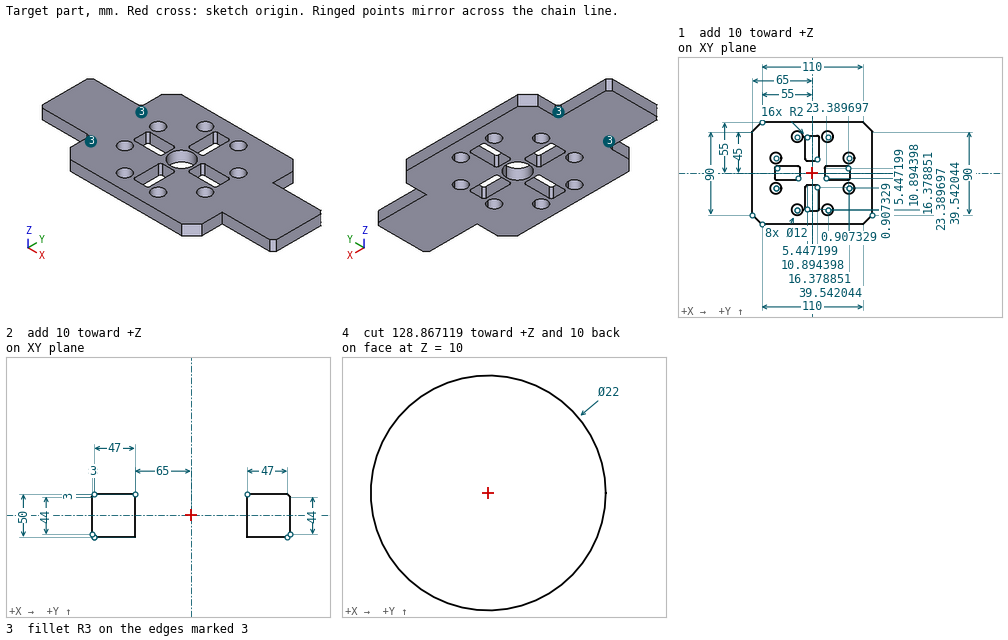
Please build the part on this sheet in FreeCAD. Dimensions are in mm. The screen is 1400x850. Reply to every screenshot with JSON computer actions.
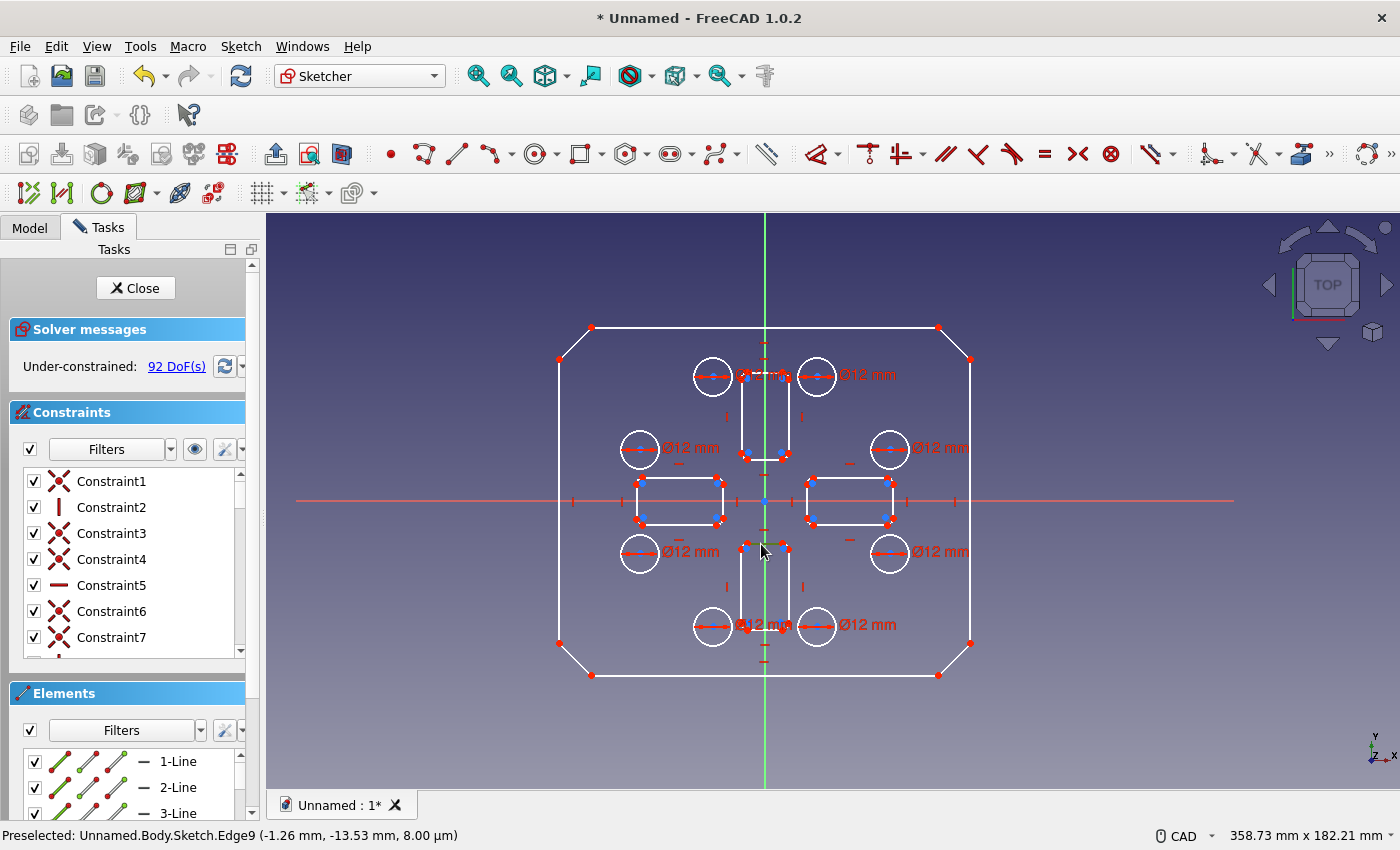
{"action": "scroll", "coordinate": [787, 545], "scroll_direction": "up", "scroll_amount": 6}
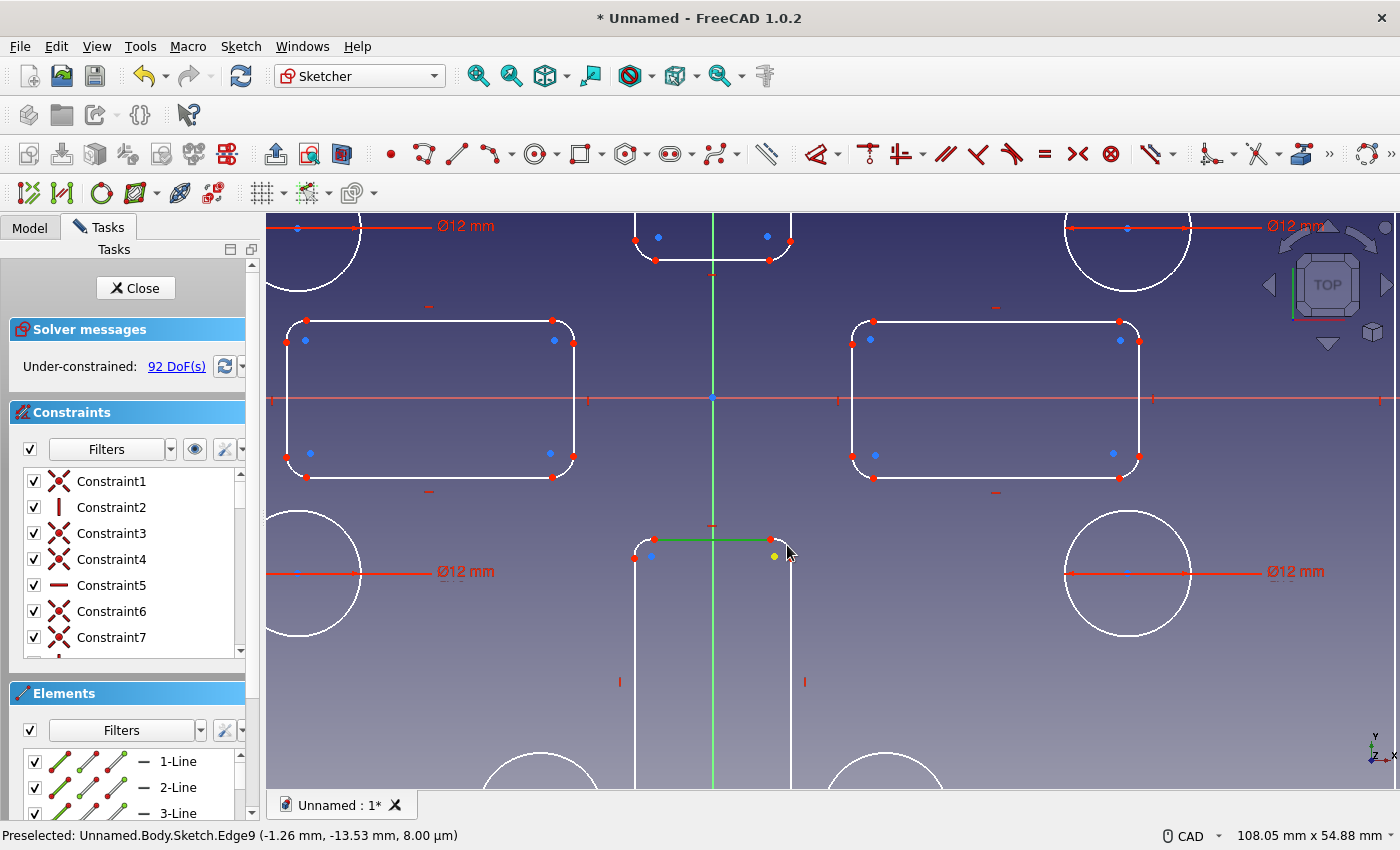
{"action": "left_click", "coordinate": [786, 544]}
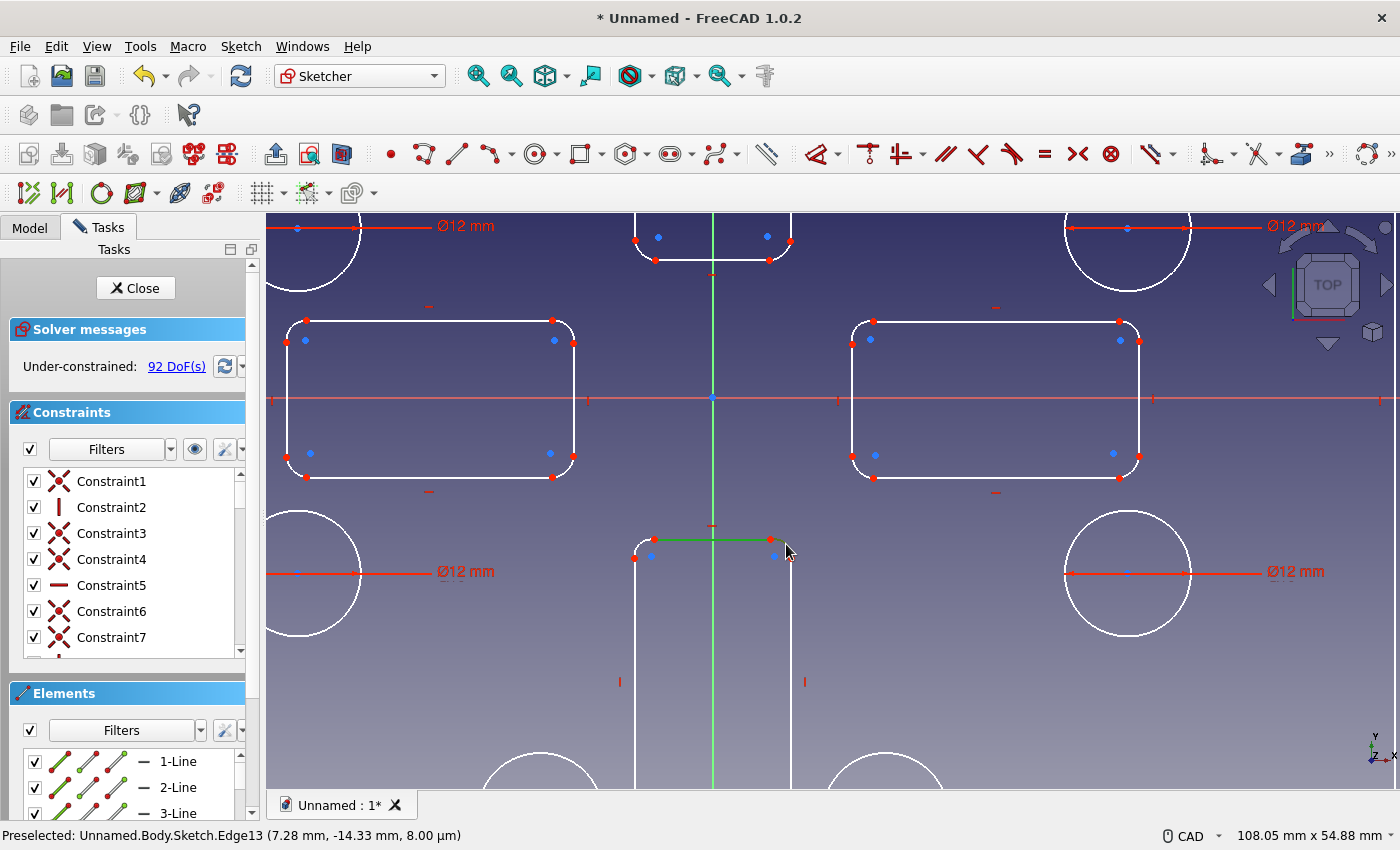
{"action": "left_click", "coordinate": [1012, 154]}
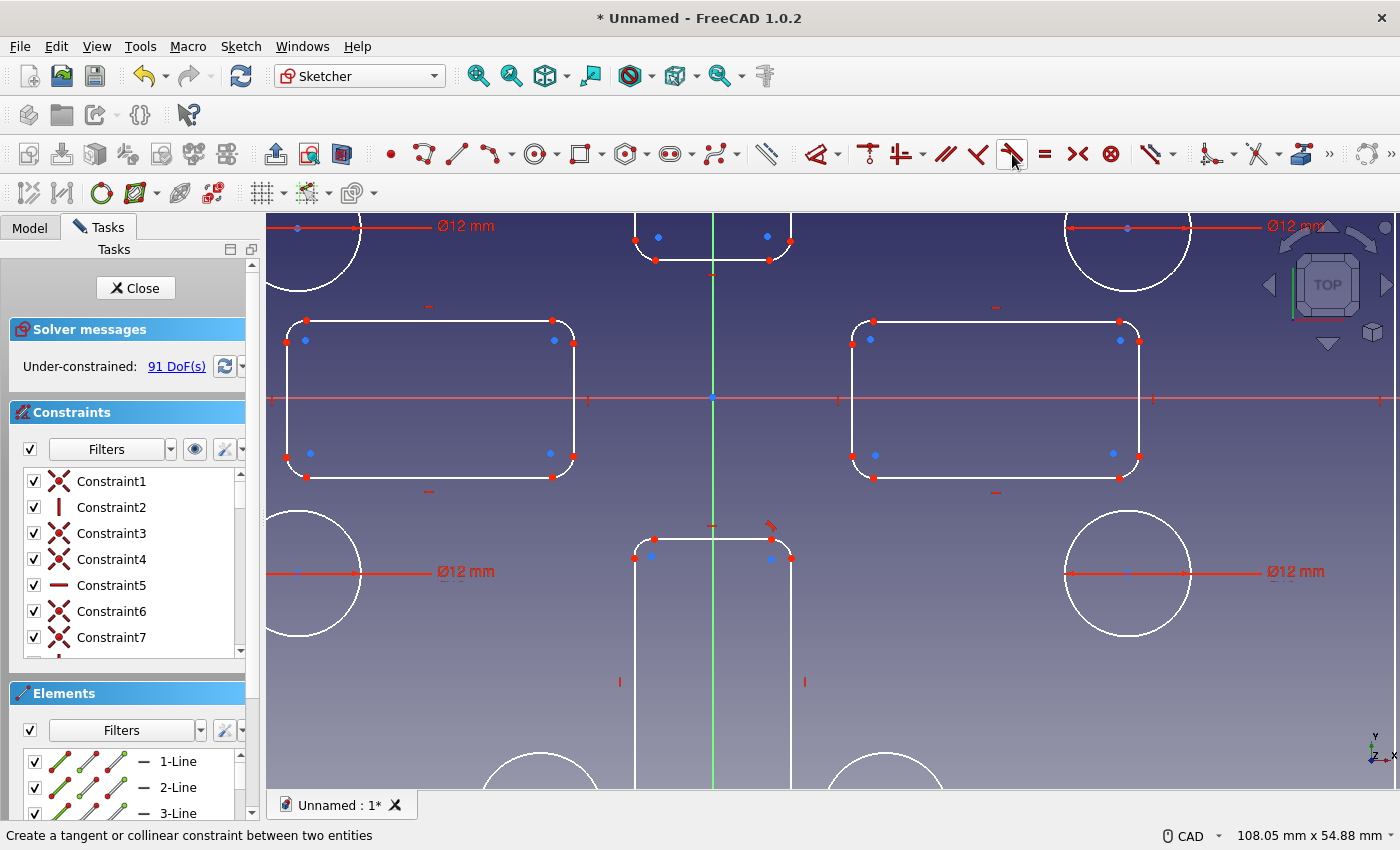
{"action": "left_click", "coordinate": [689, 539]}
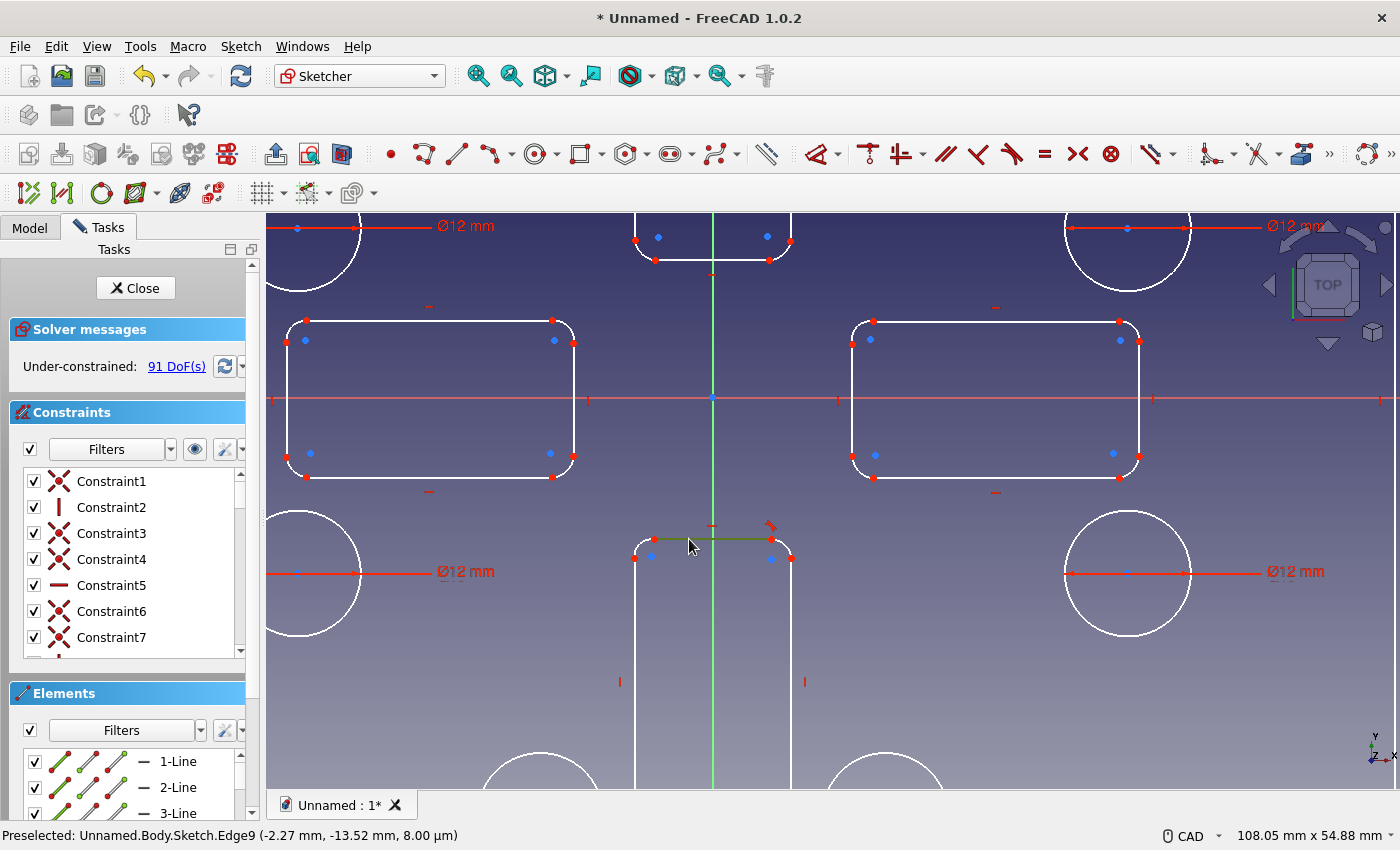
{"action": "scroll", "coordinate": [645, 541], "scroll_direction": "up", "scroll_amount": 2}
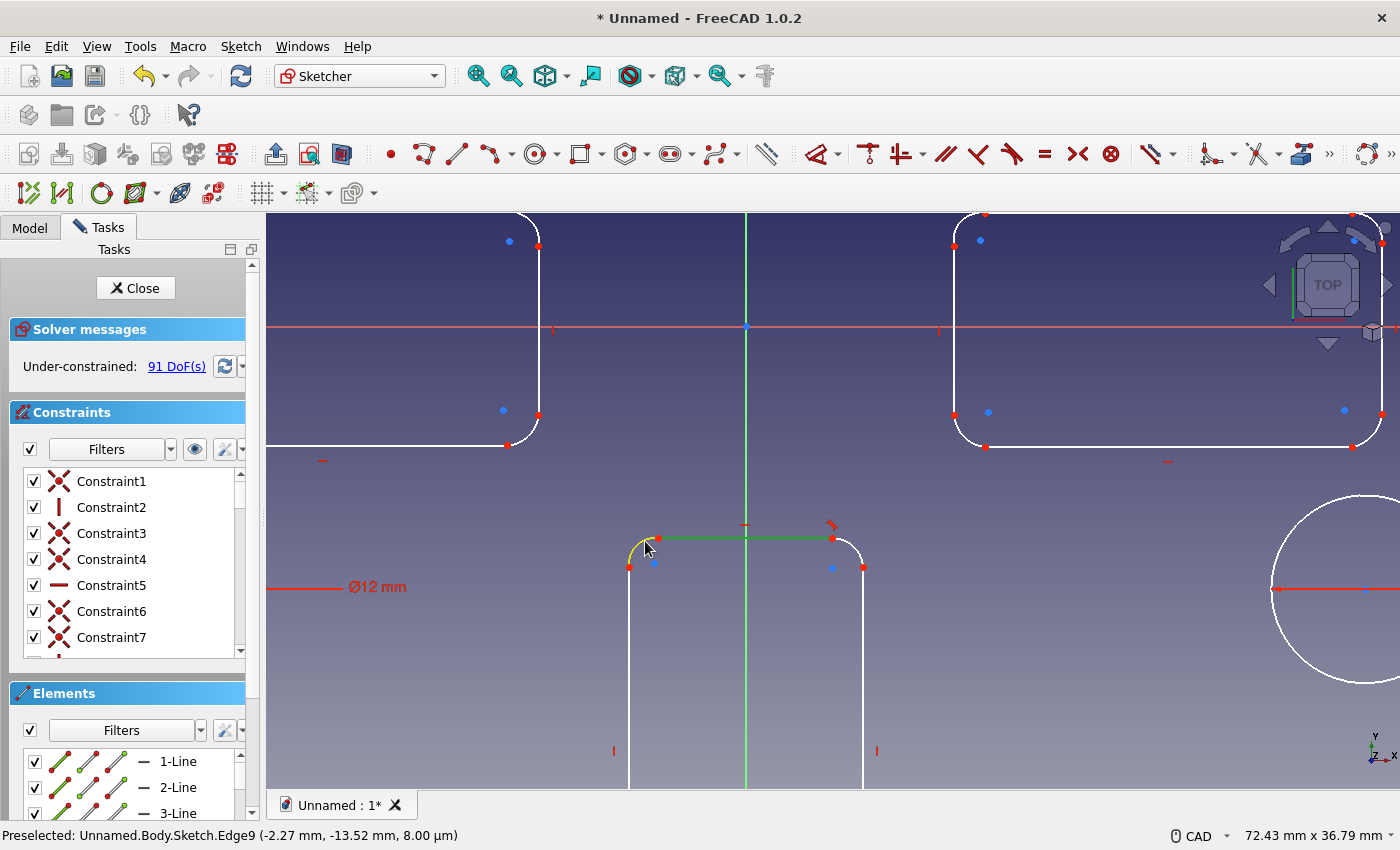
{"action": "left_click", "coordinate": [645, 540]}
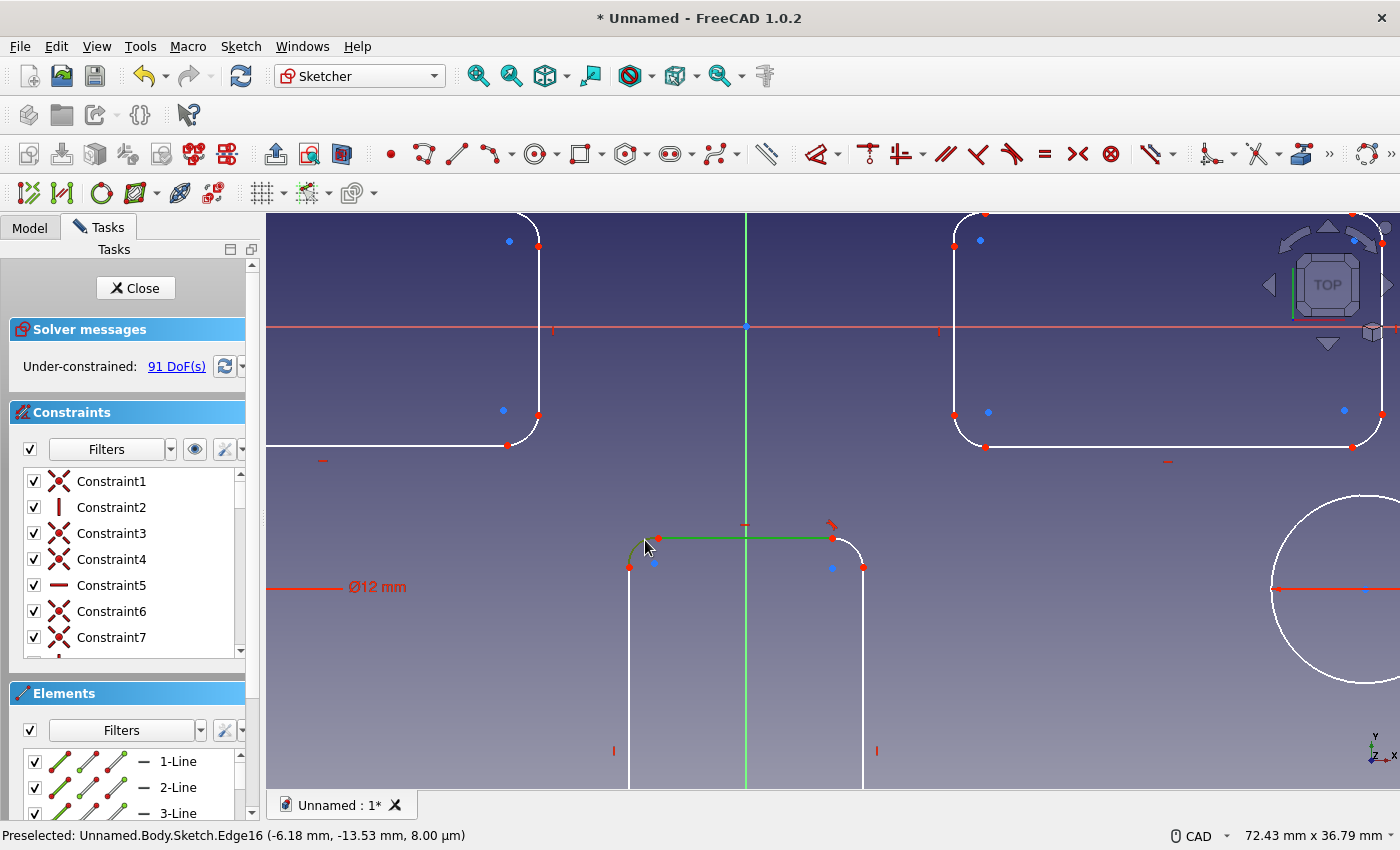
{"action": "left_click", "coordinate": [1012, 154]}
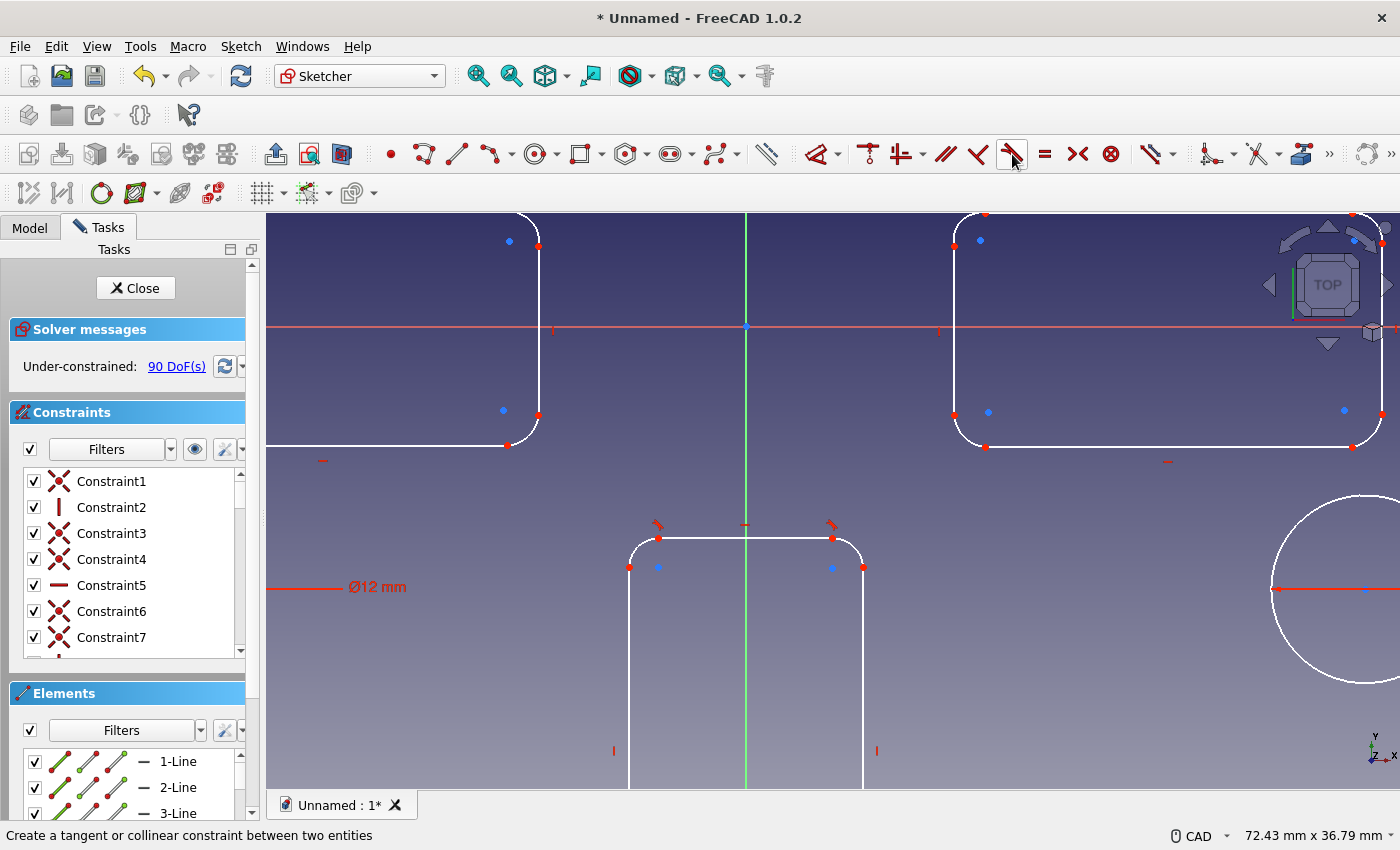
{"action": "scroll", "coordinate": [769, 545], "scroll_direction": "down", "scroll_amount": 8}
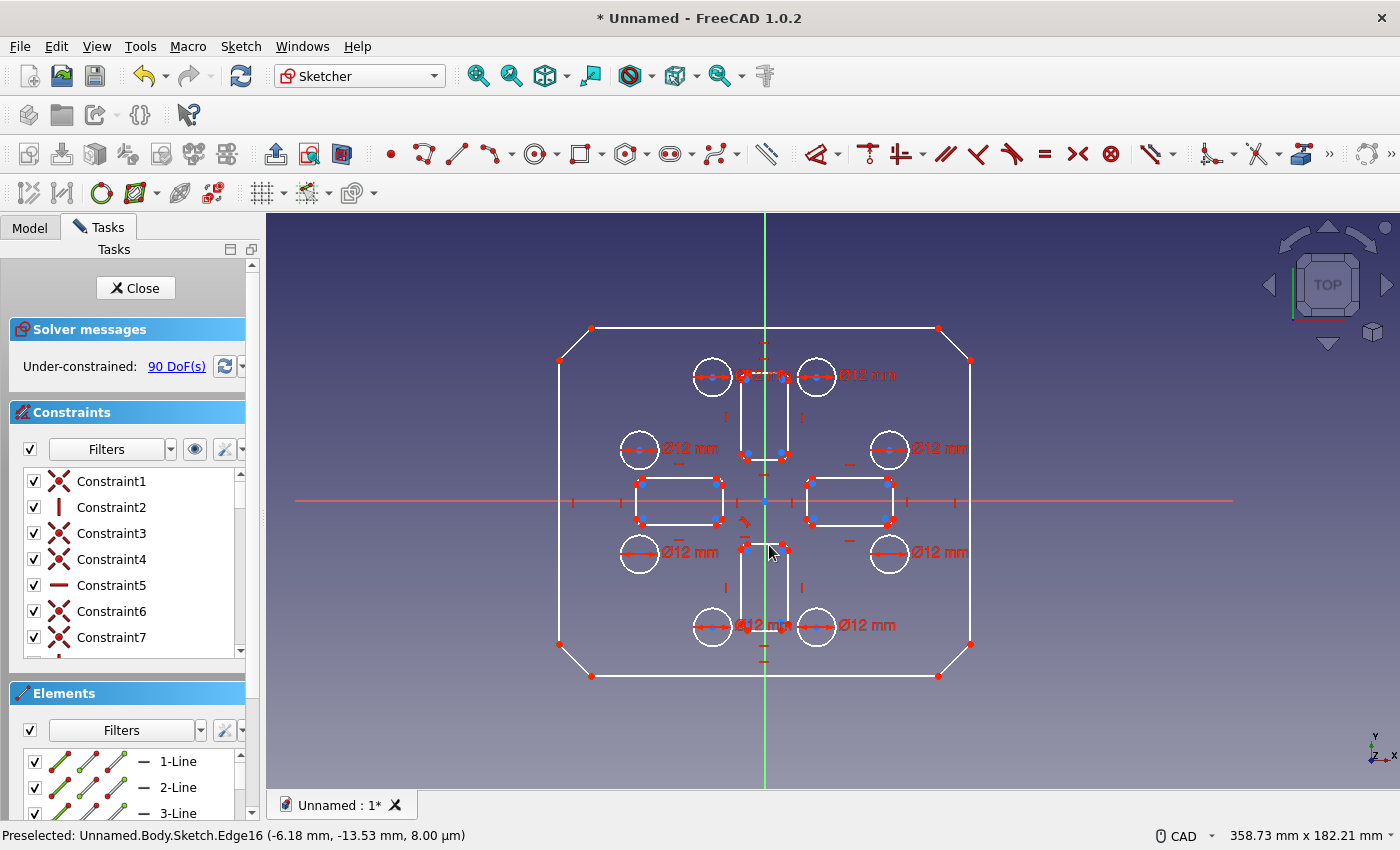
{"action": "left_click", "coordinate": [788, 572]}